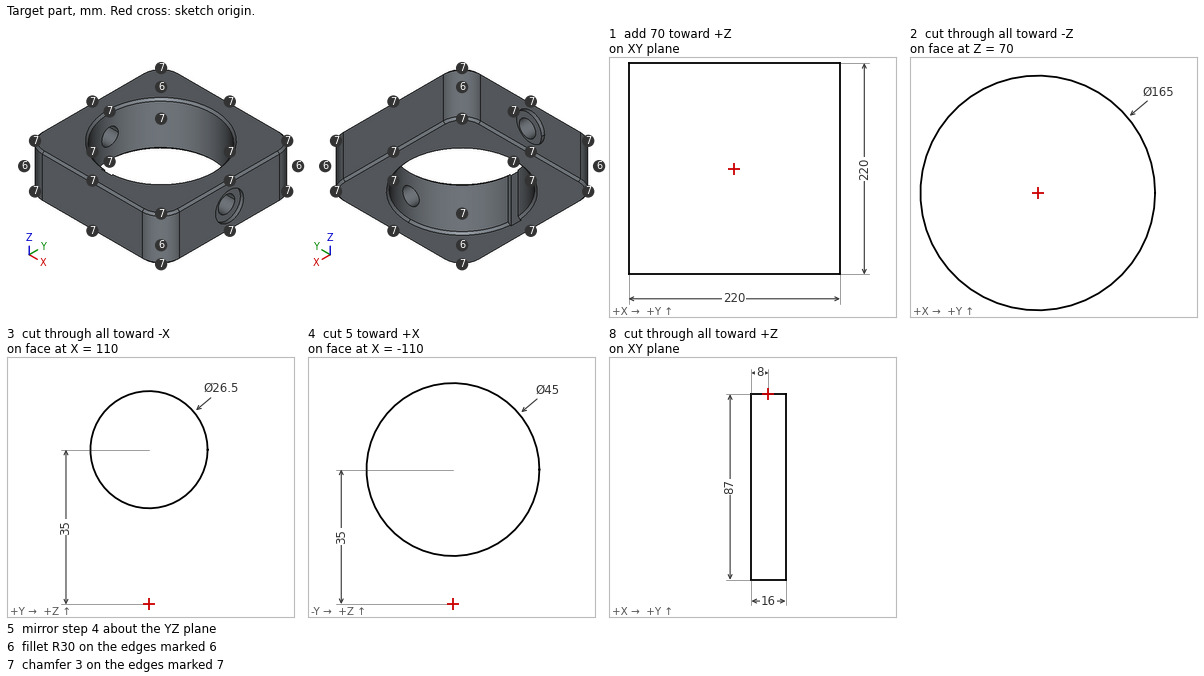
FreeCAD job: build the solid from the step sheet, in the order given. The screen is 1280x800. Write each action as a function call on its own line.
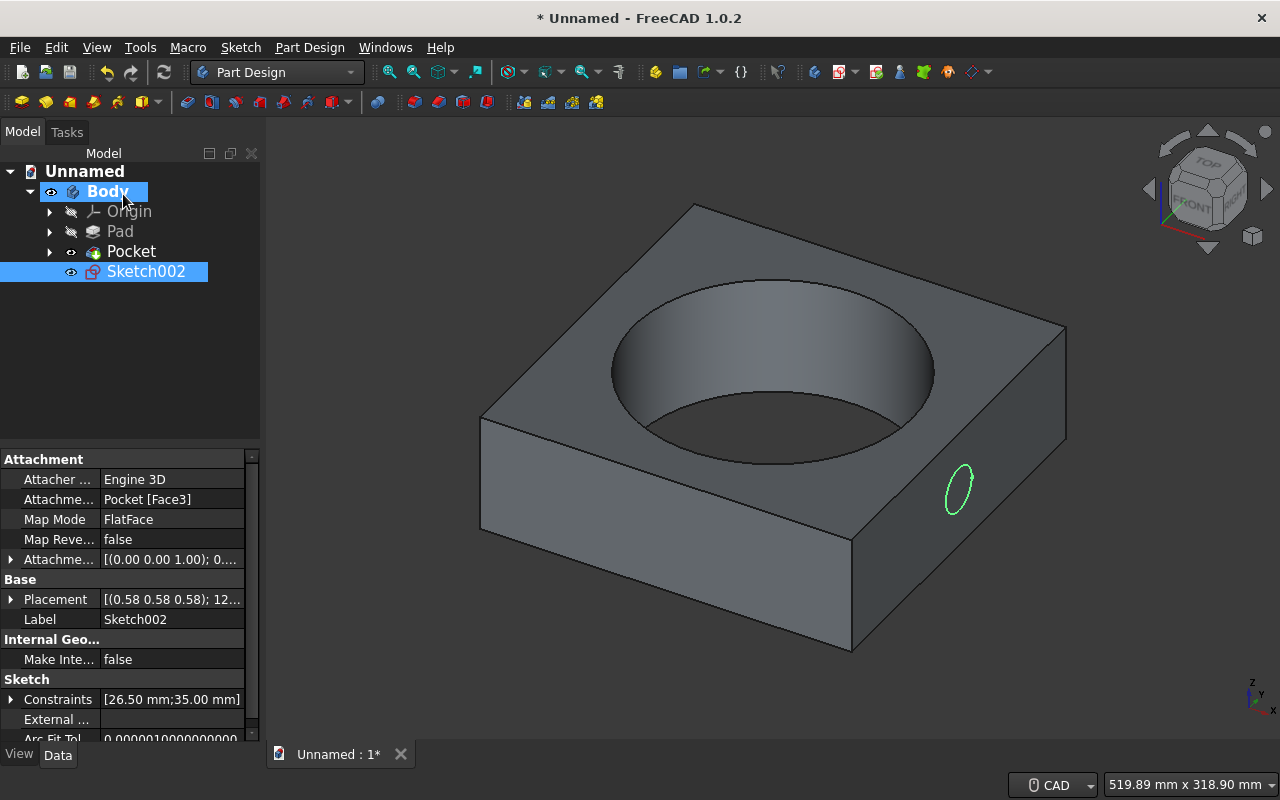
click(188, 102)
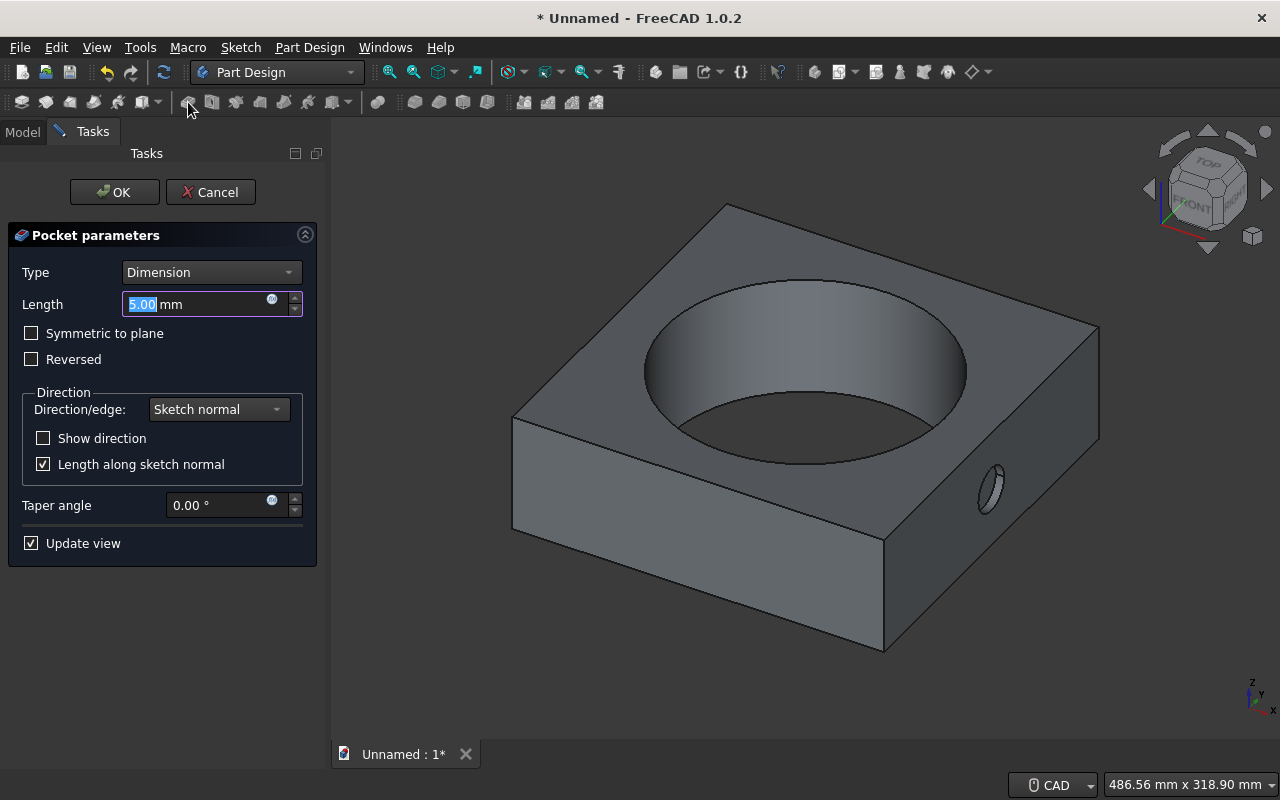
click(212, 272)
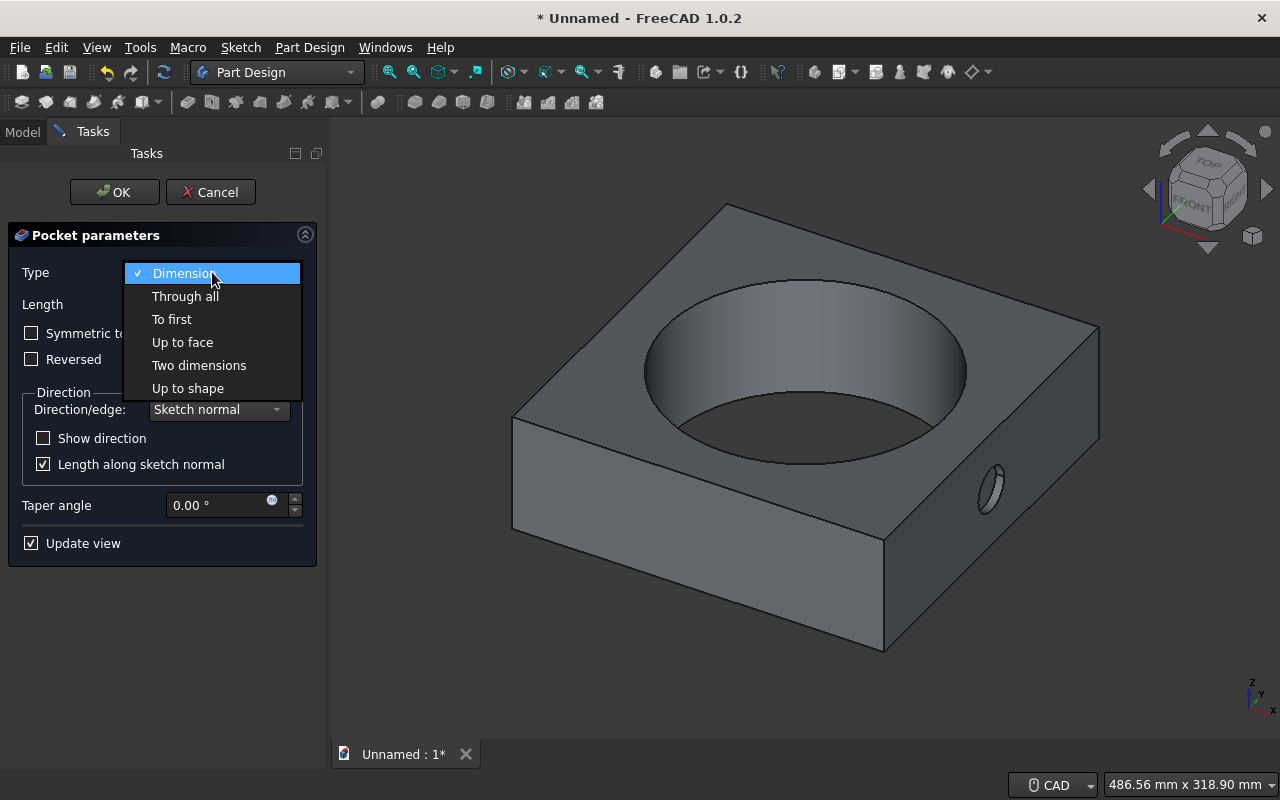
click(212, 296)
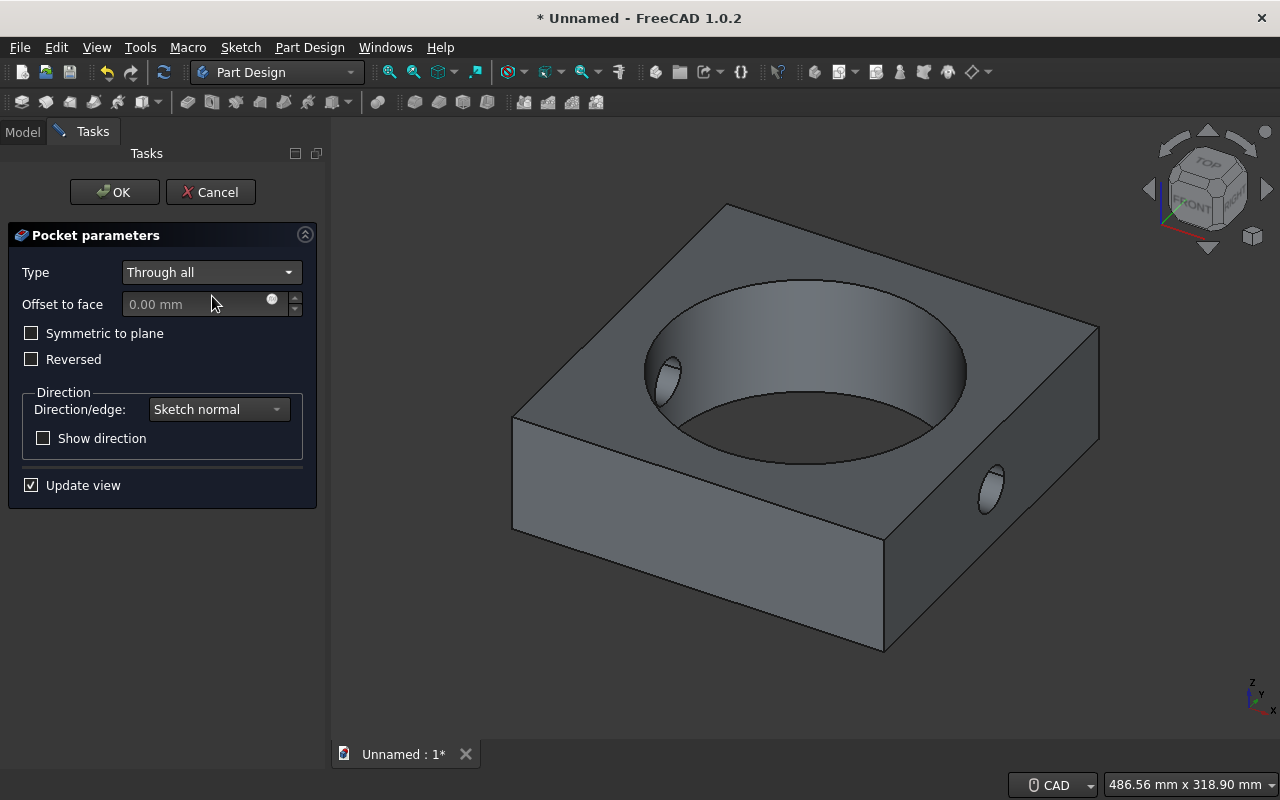
click(115, 192)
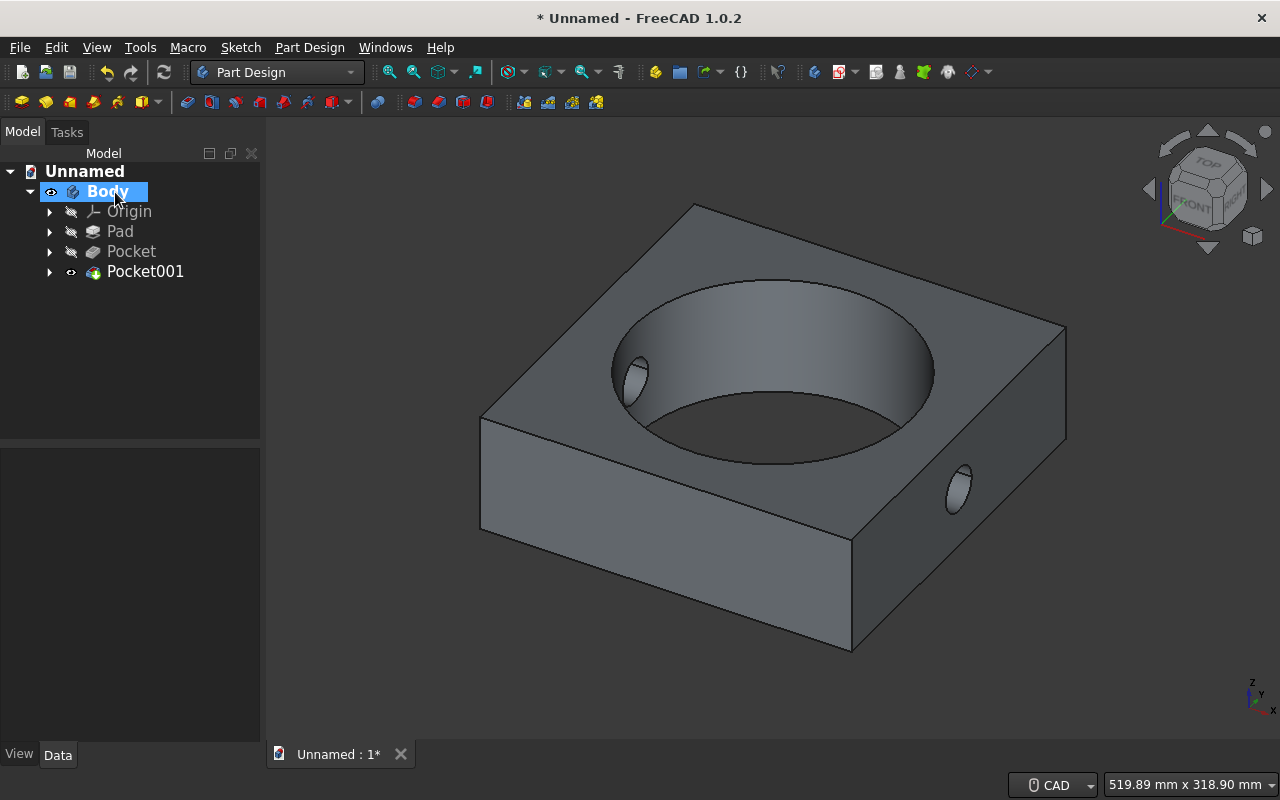
key(6)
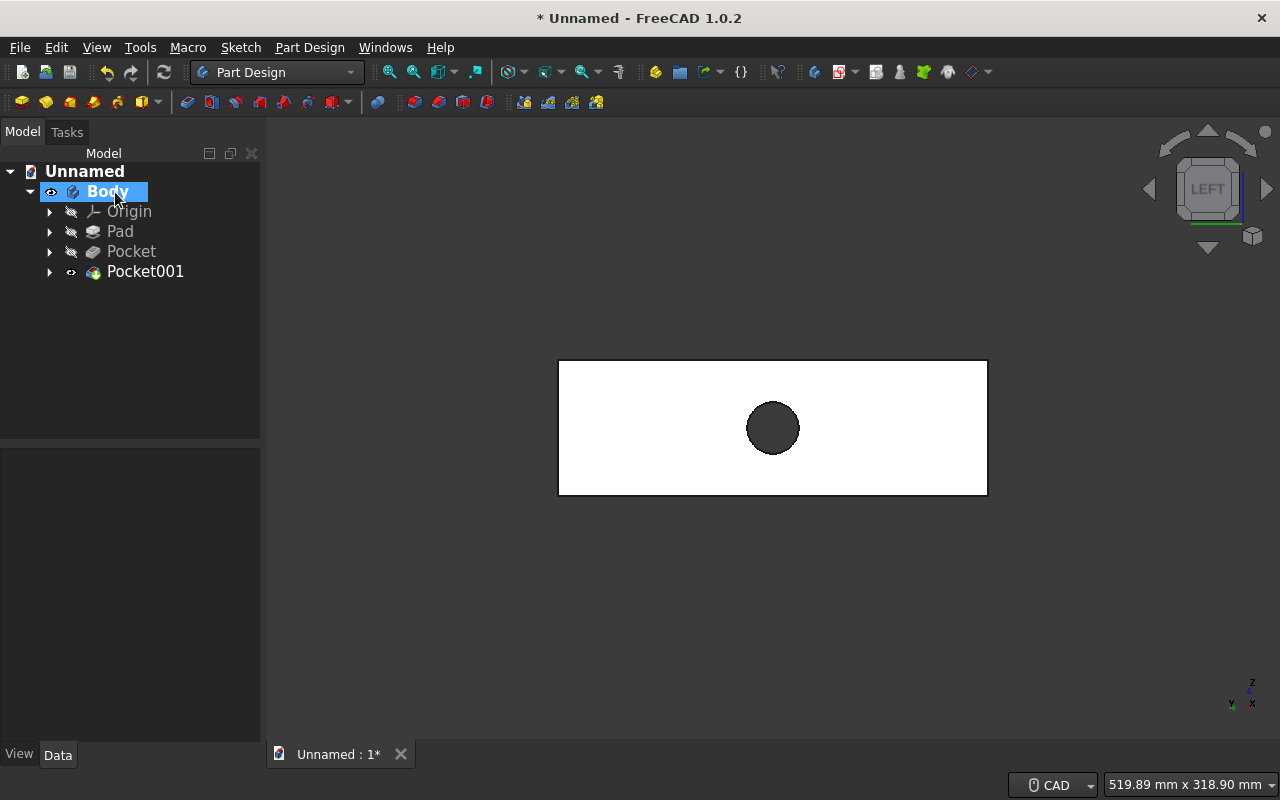
key(v)
key(f)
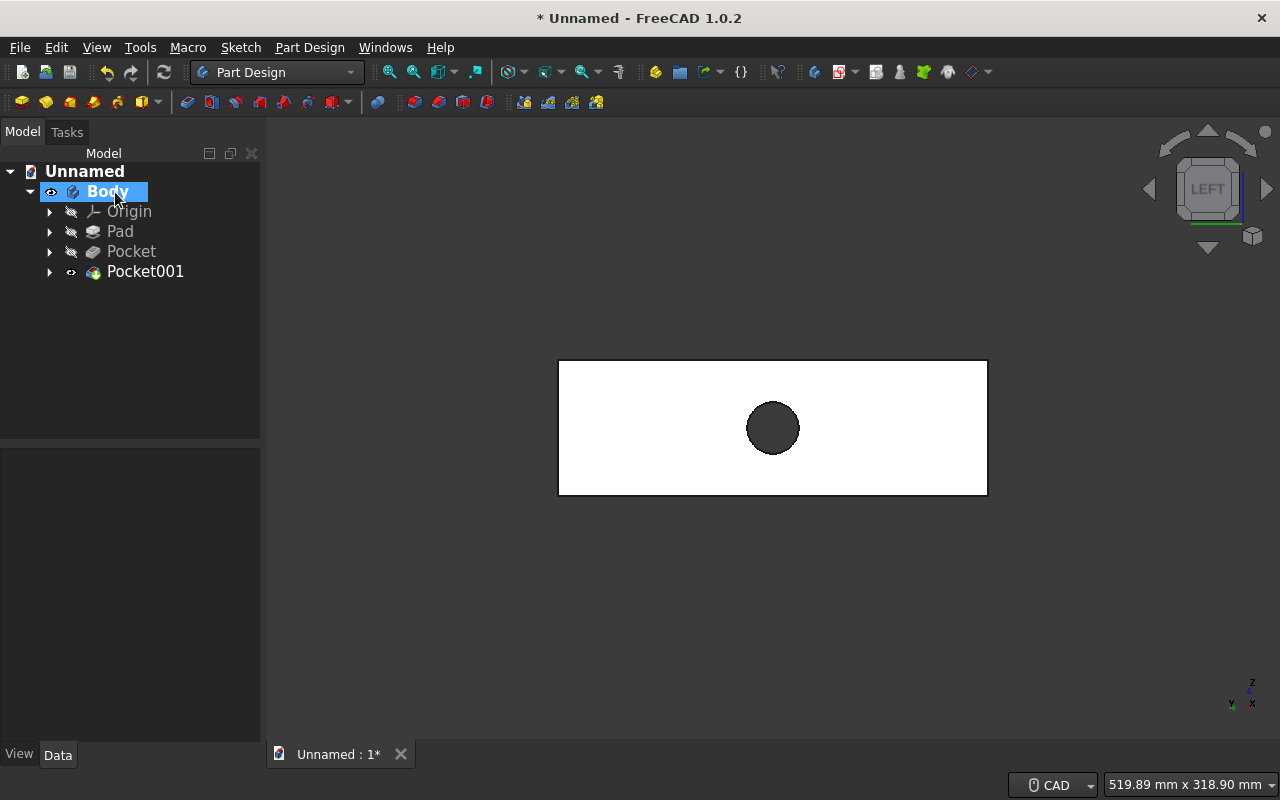
click(650, 427)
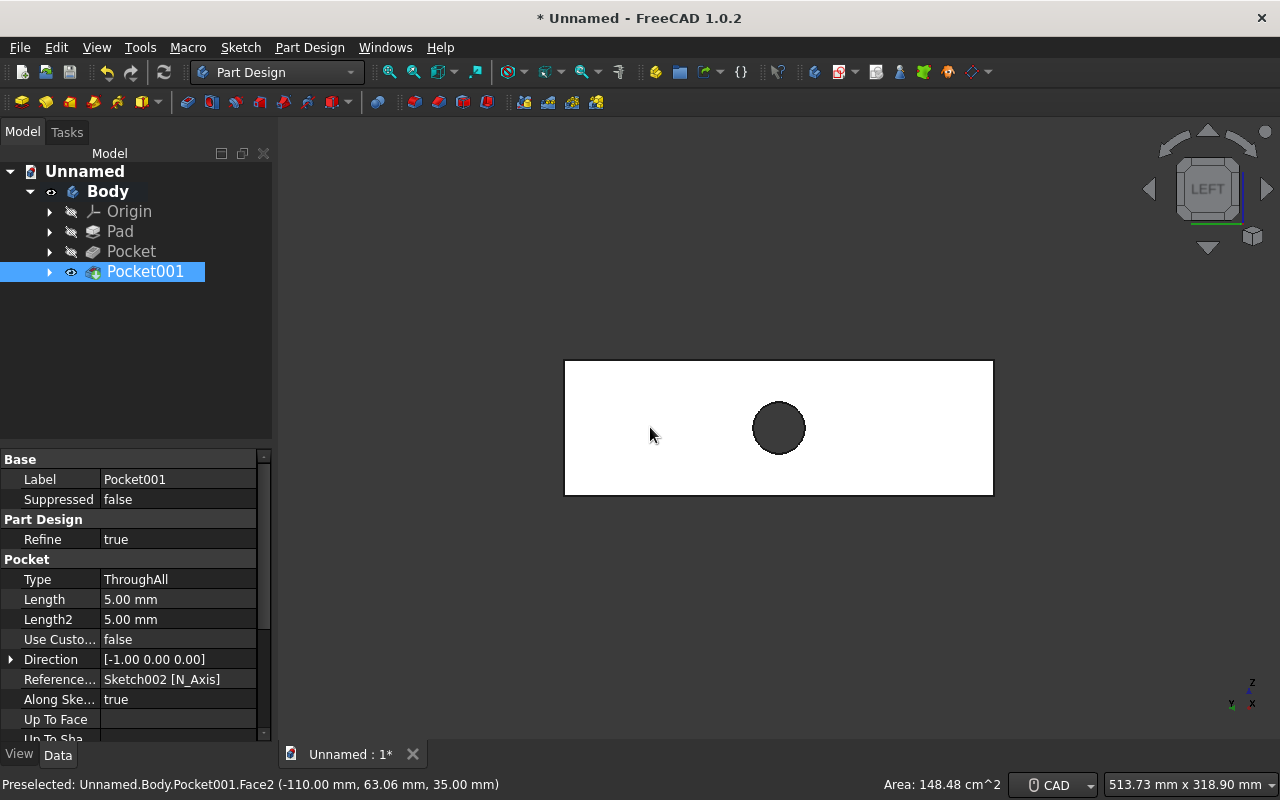
click(840, 72)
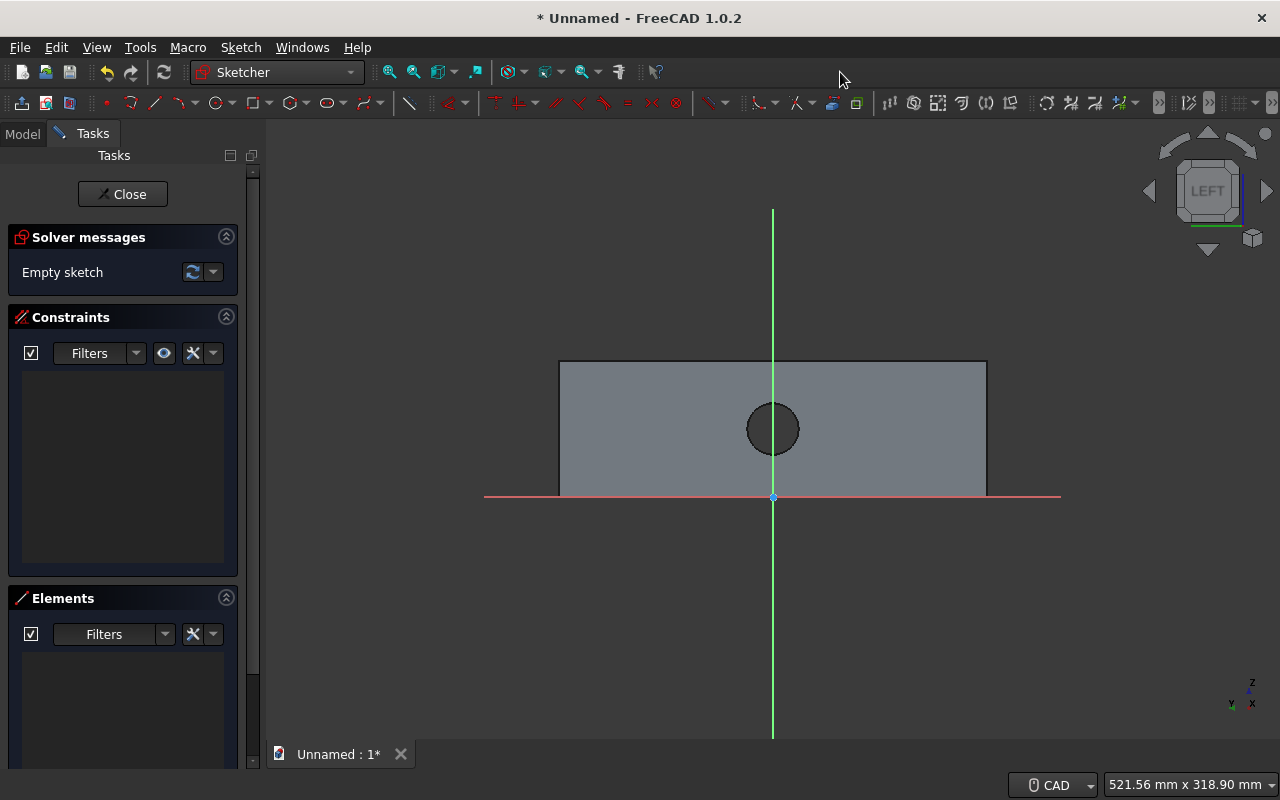
scroll(803, 446, up, 6)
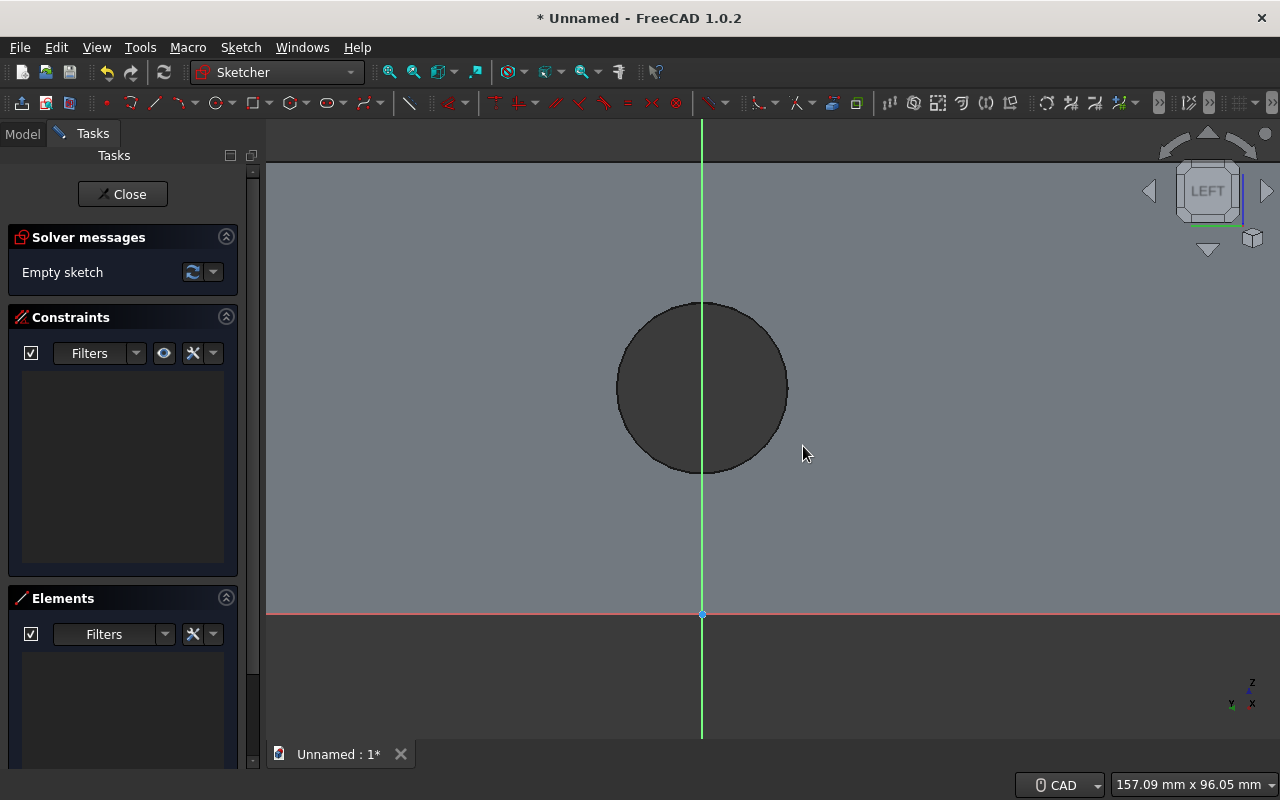
key(g)
key(c)